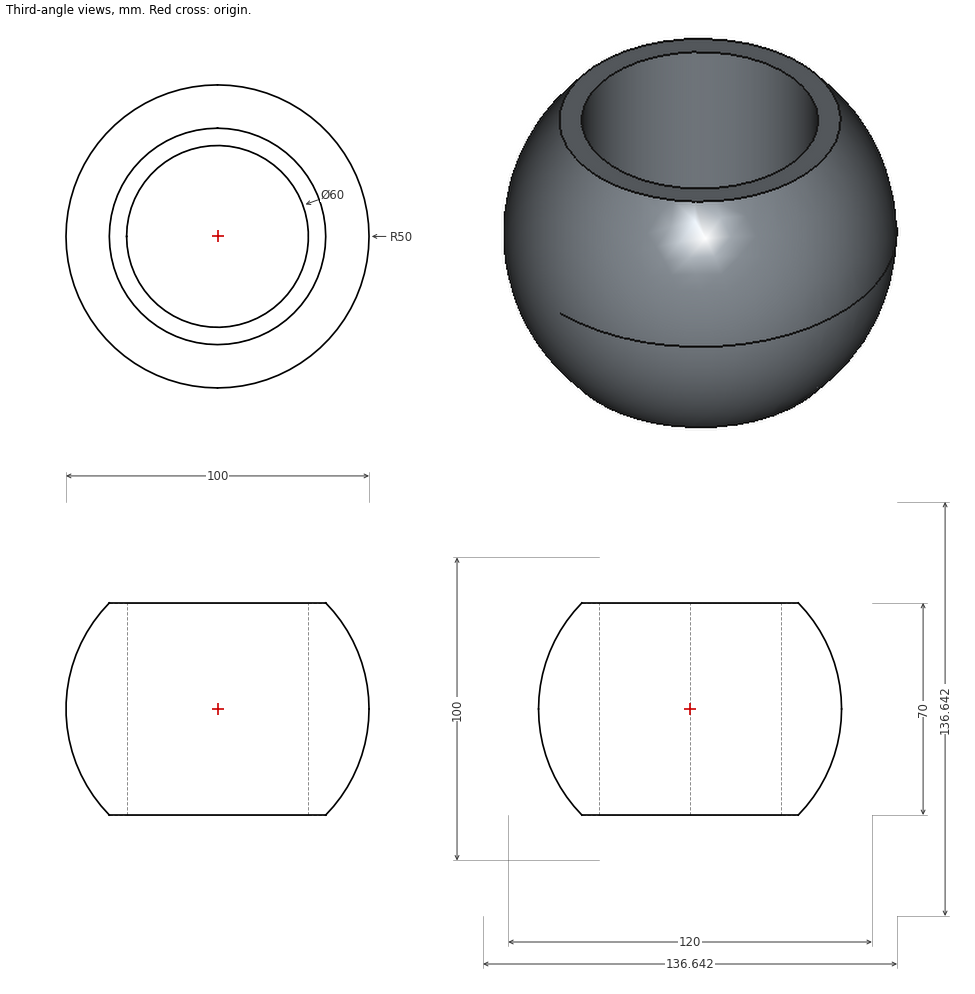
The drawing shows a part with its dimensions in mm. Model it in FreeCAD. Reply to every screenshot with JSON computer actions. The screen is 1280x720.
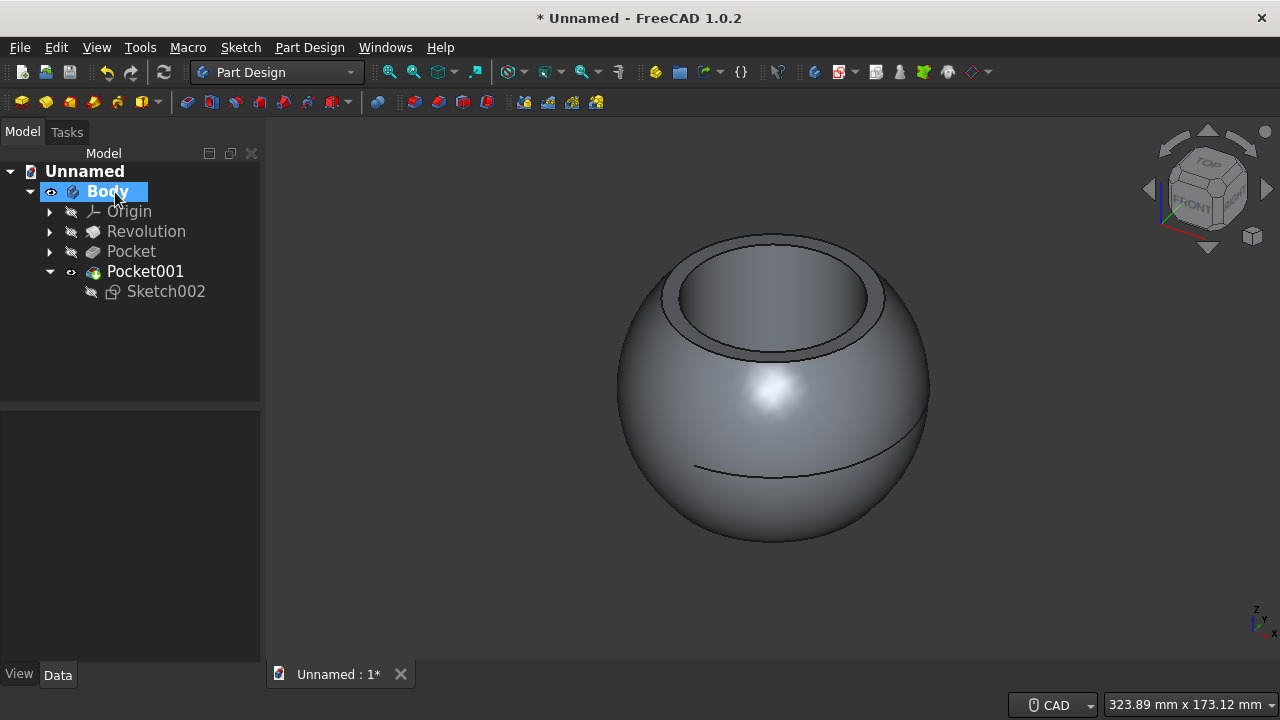
{"action": "key", "text": "0"}